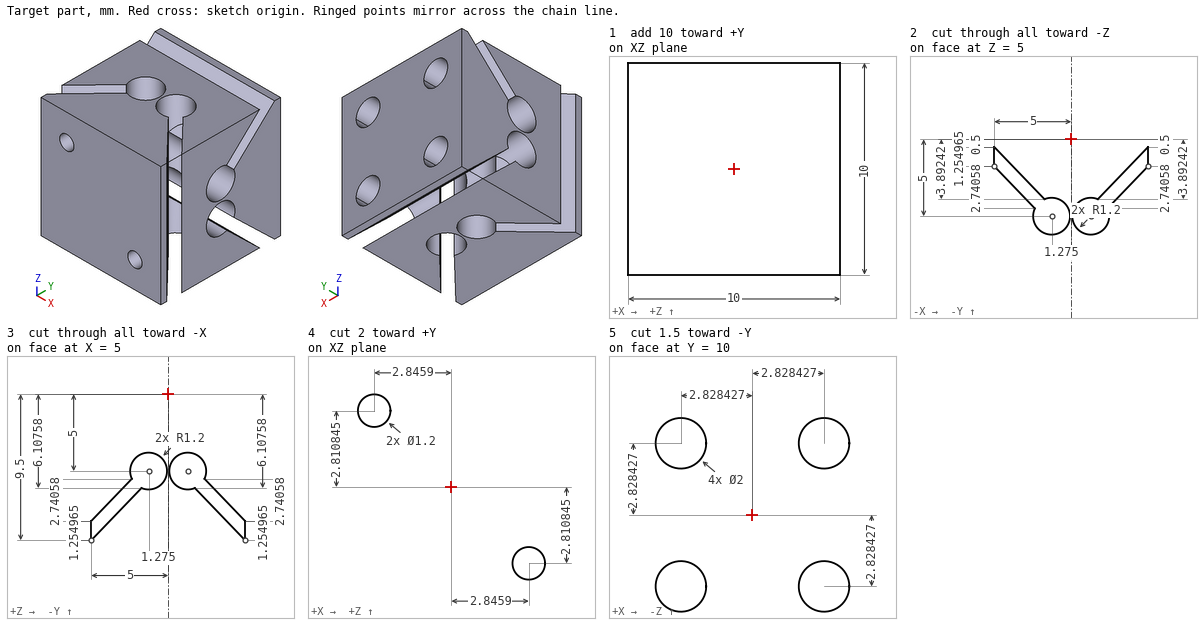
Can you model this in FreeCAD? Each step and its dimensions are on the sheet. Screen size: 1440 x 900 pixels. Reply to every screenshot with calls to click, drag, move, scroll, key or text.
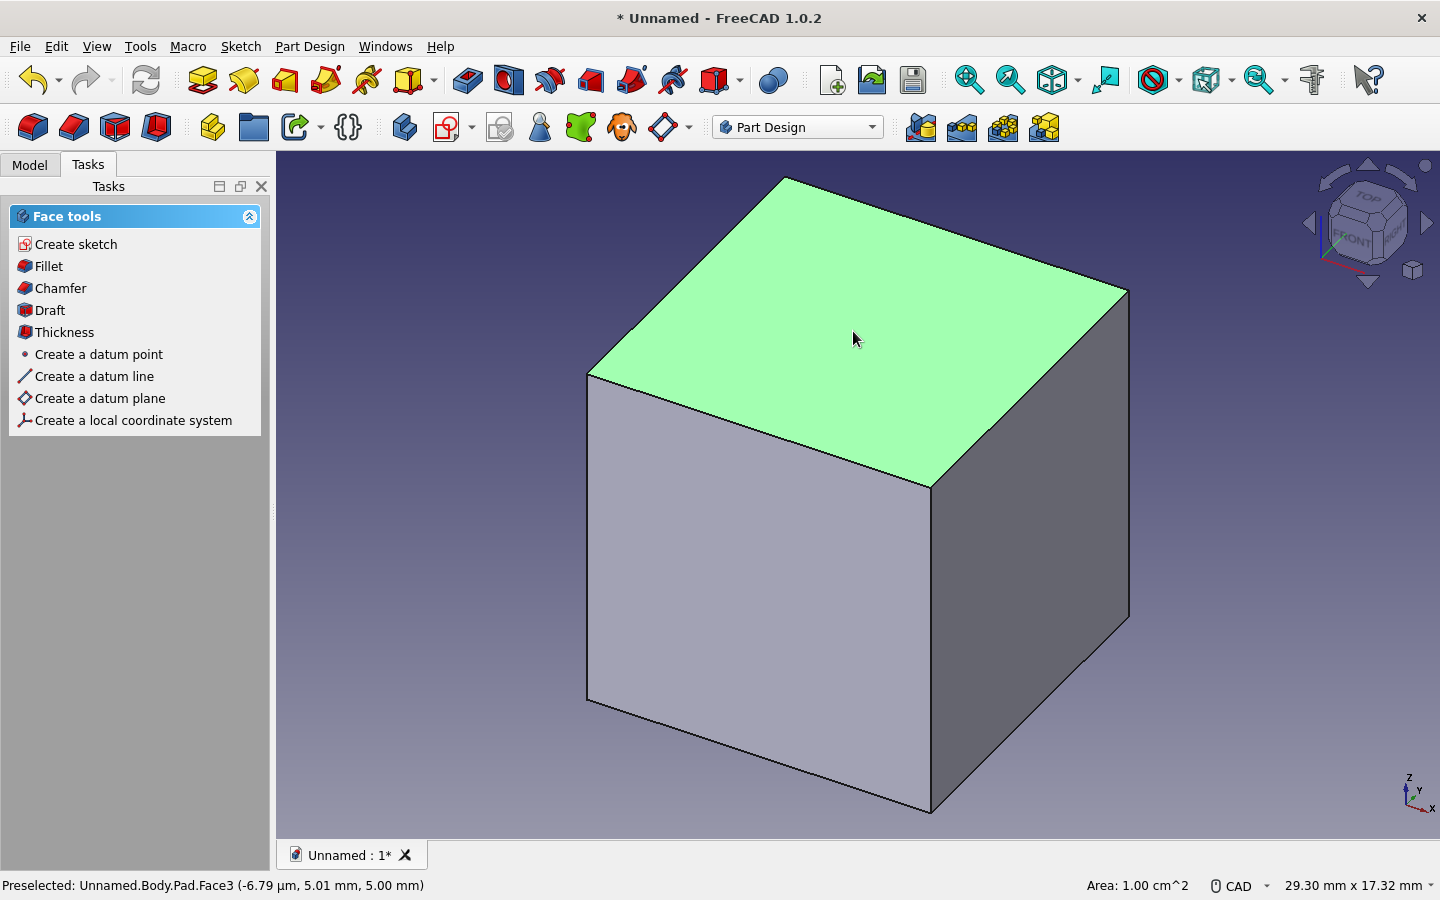
click(446, 128)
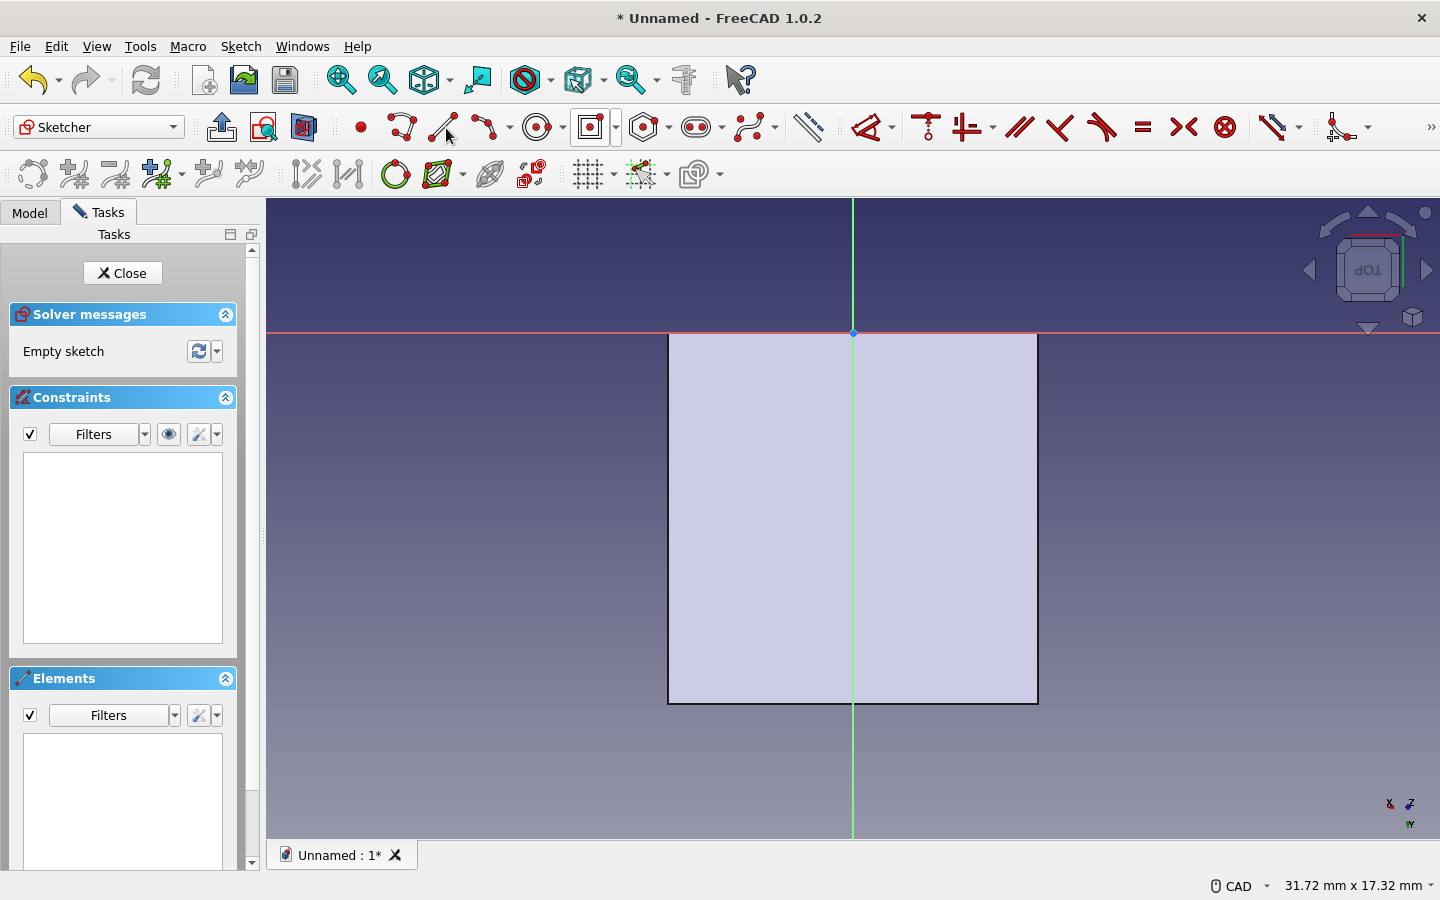
scroll(936, 349, up, 3)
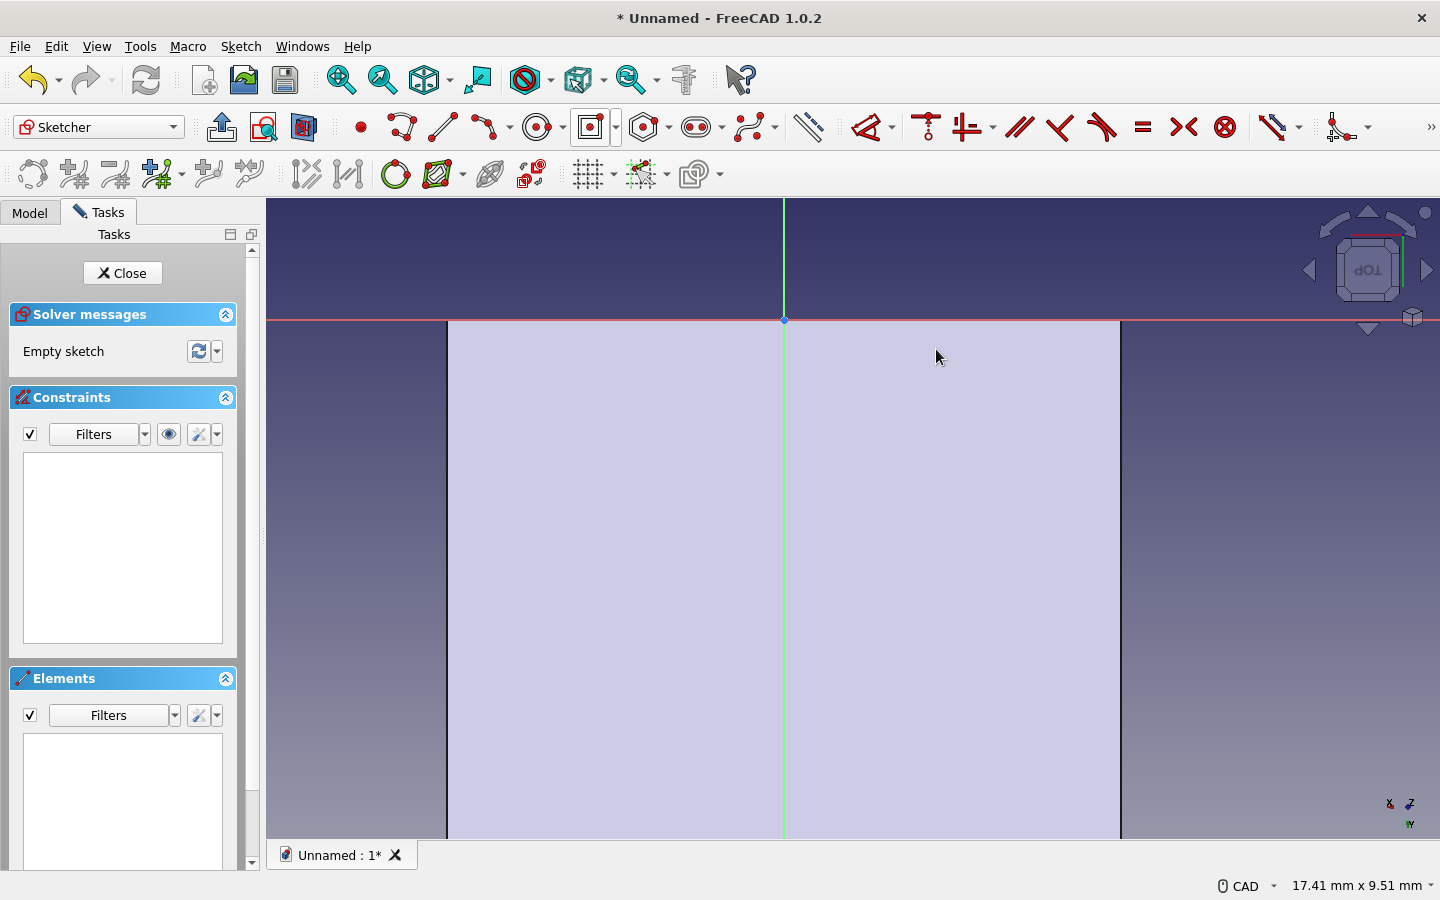
click(402, 128)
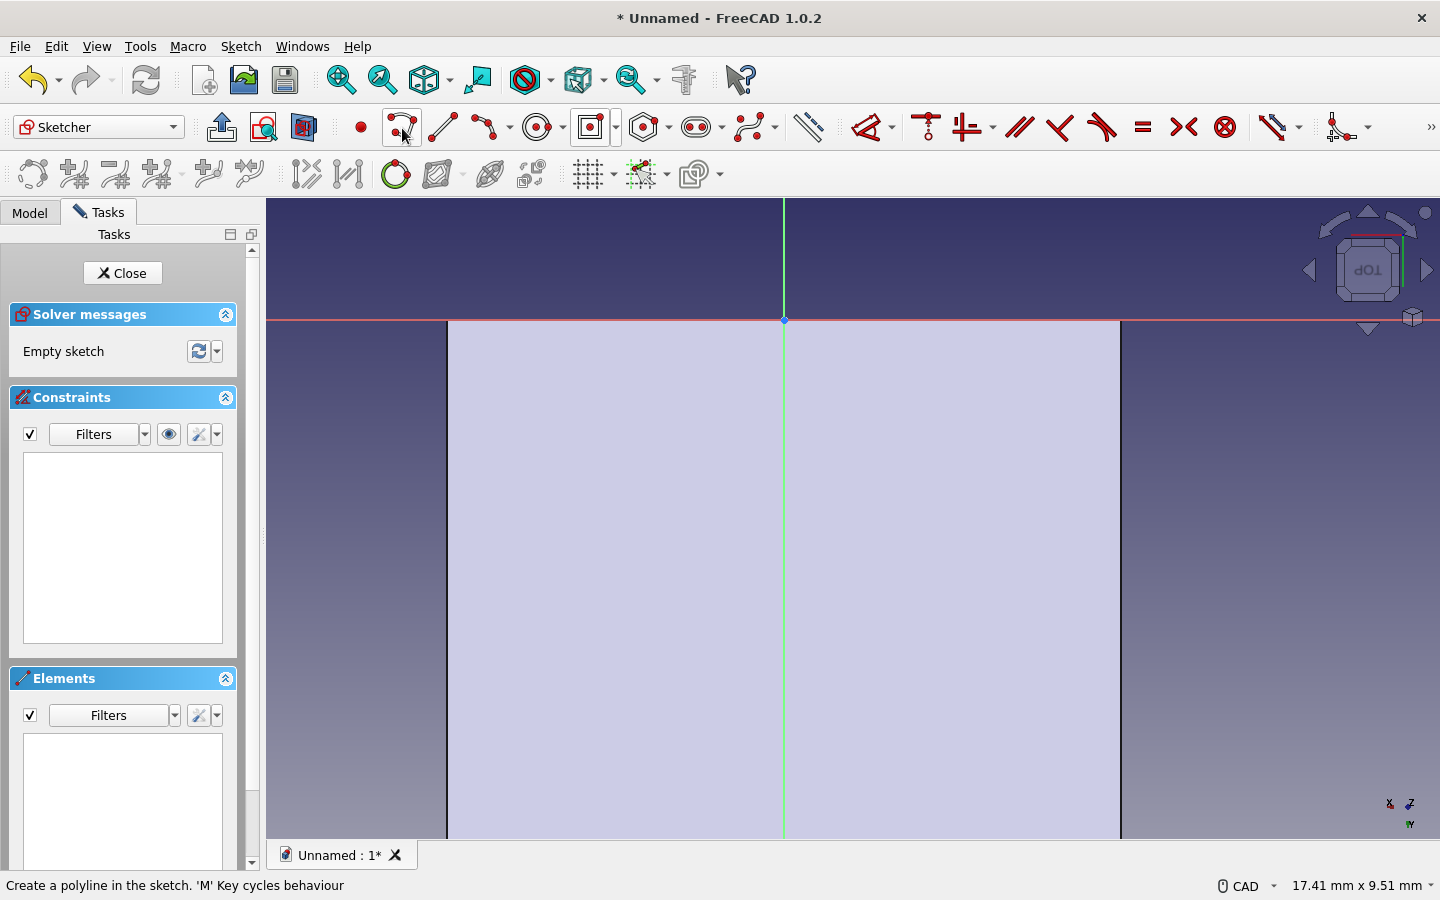
click(667, 583)
click(447, 354)
click(447, 439)
click(625, 624)
right_click(625, 624)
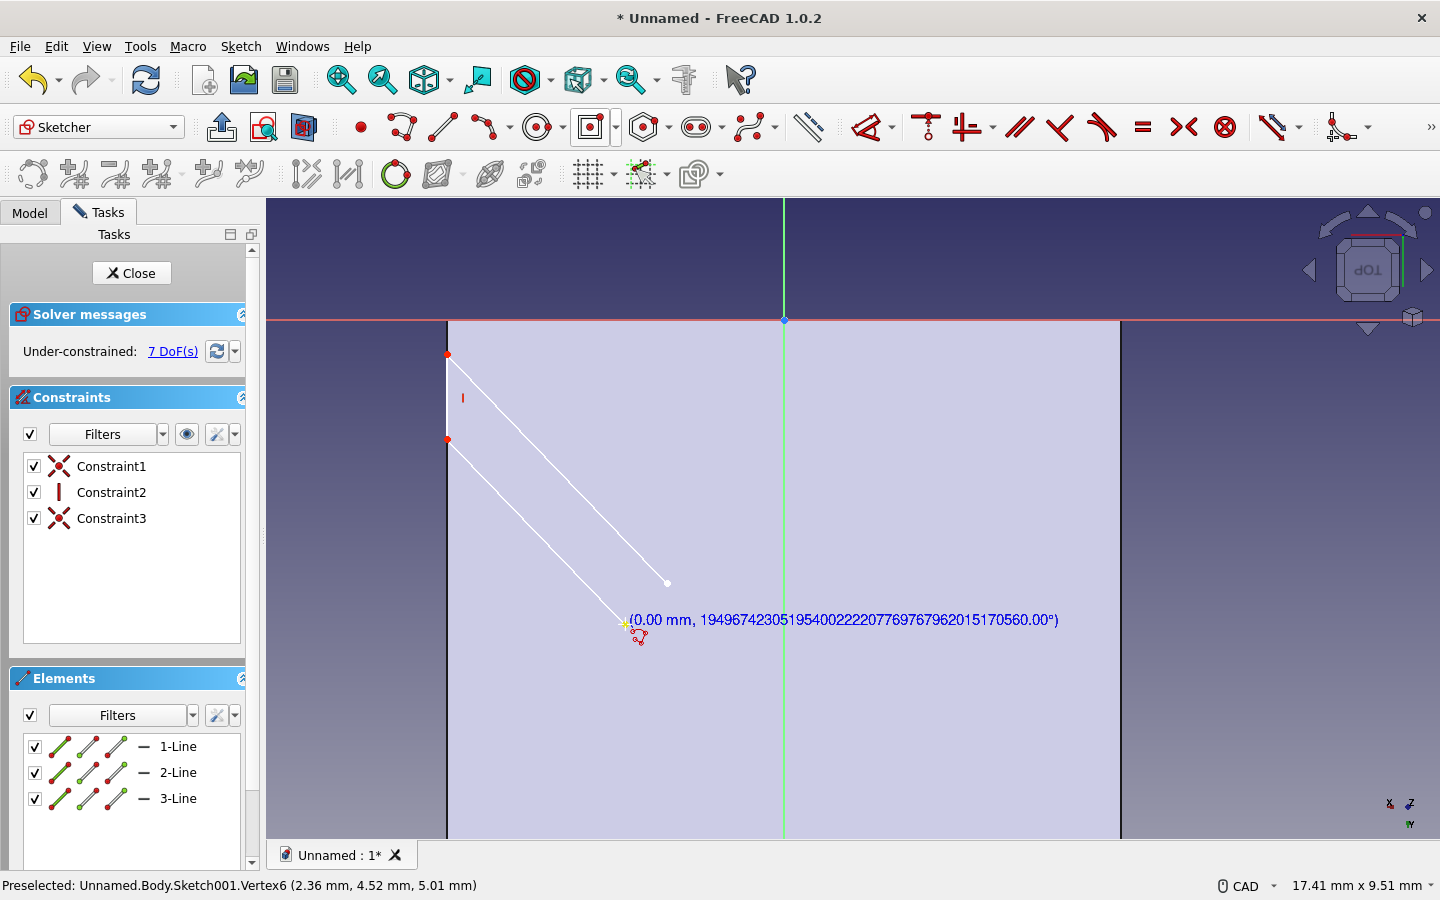
click(484, 128)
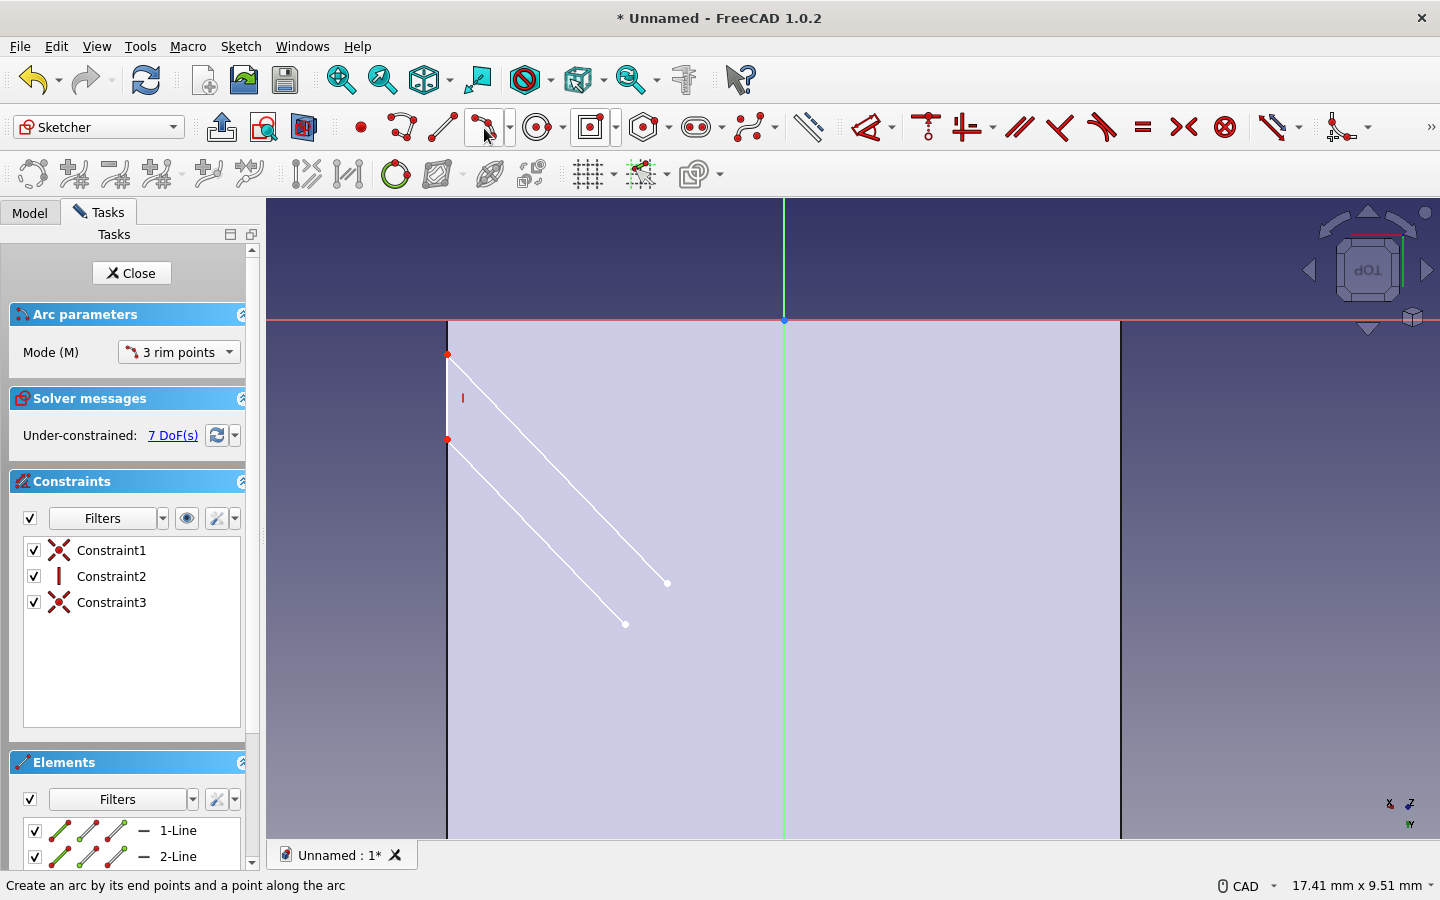
click(625, 625)
click(667, 584)
click(754, 716)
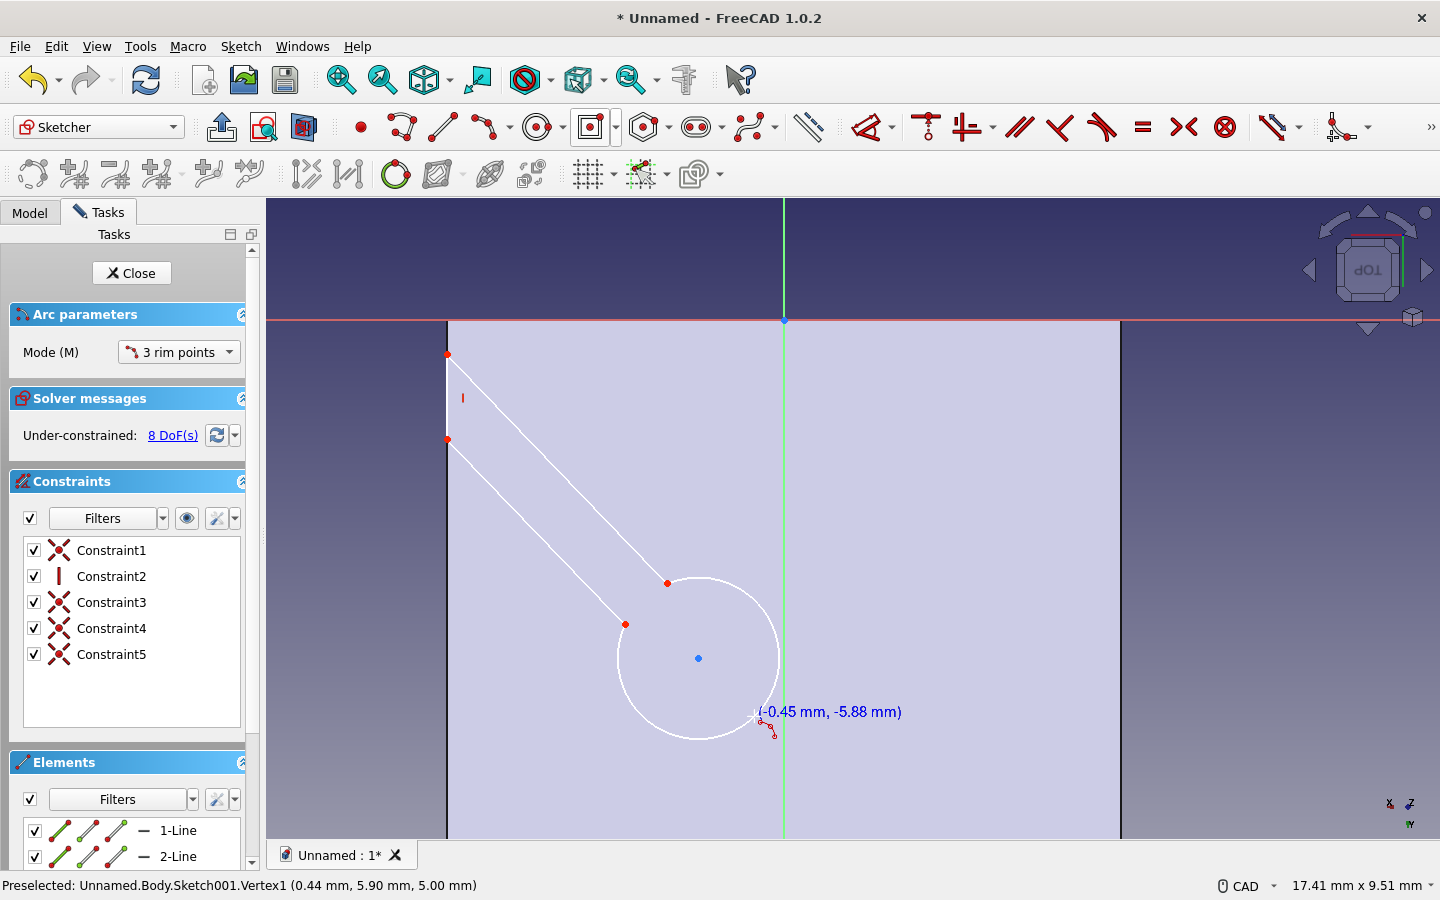
click(402, 128)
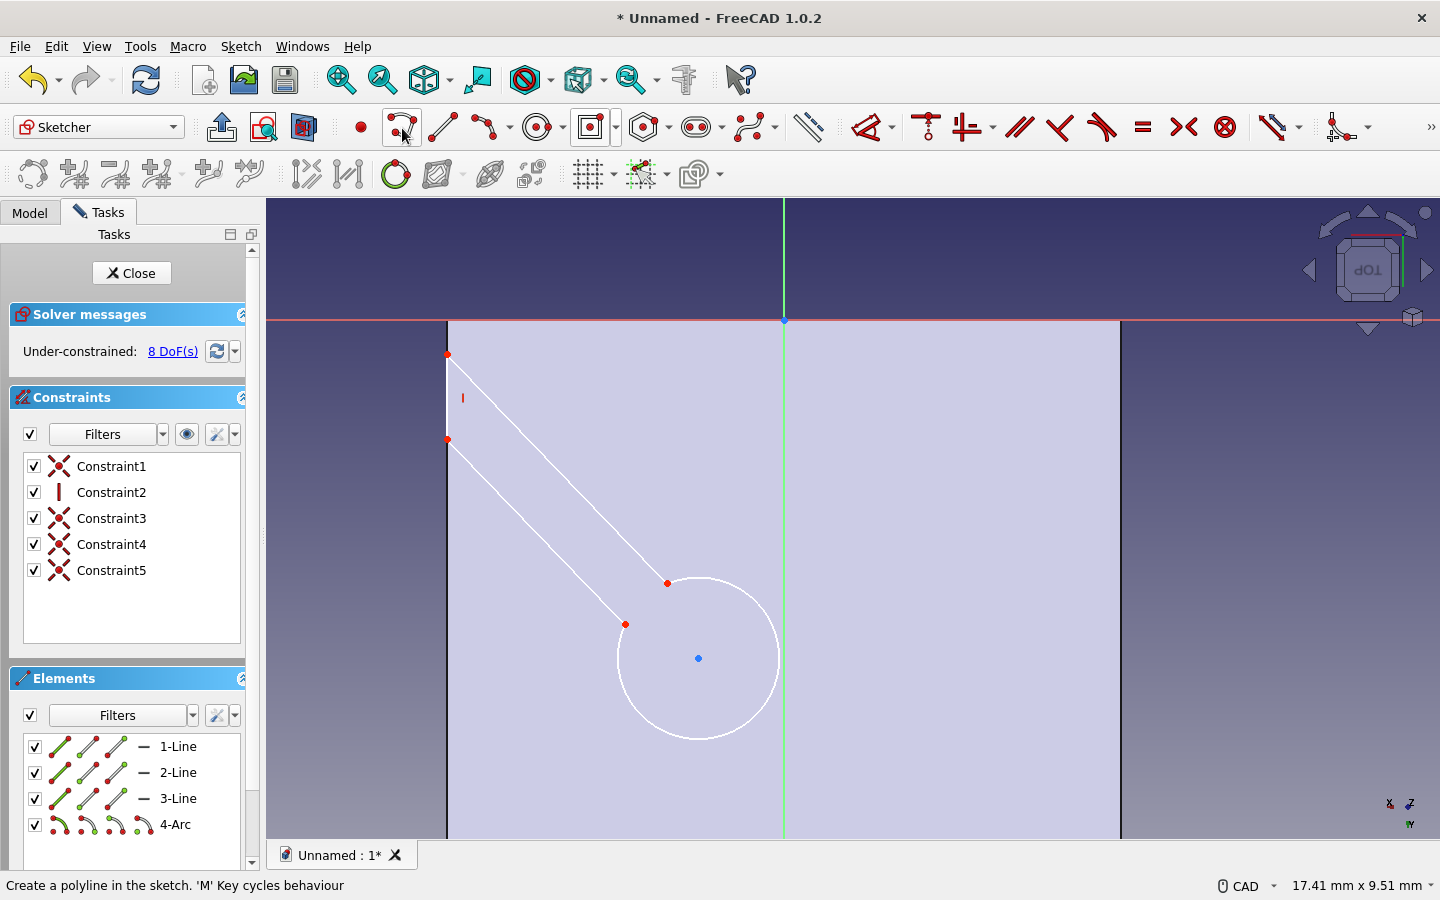
click(944, 624)
click(1121, 439)
click(1121, 354)
click(901, 583)
right_click(901, 583)